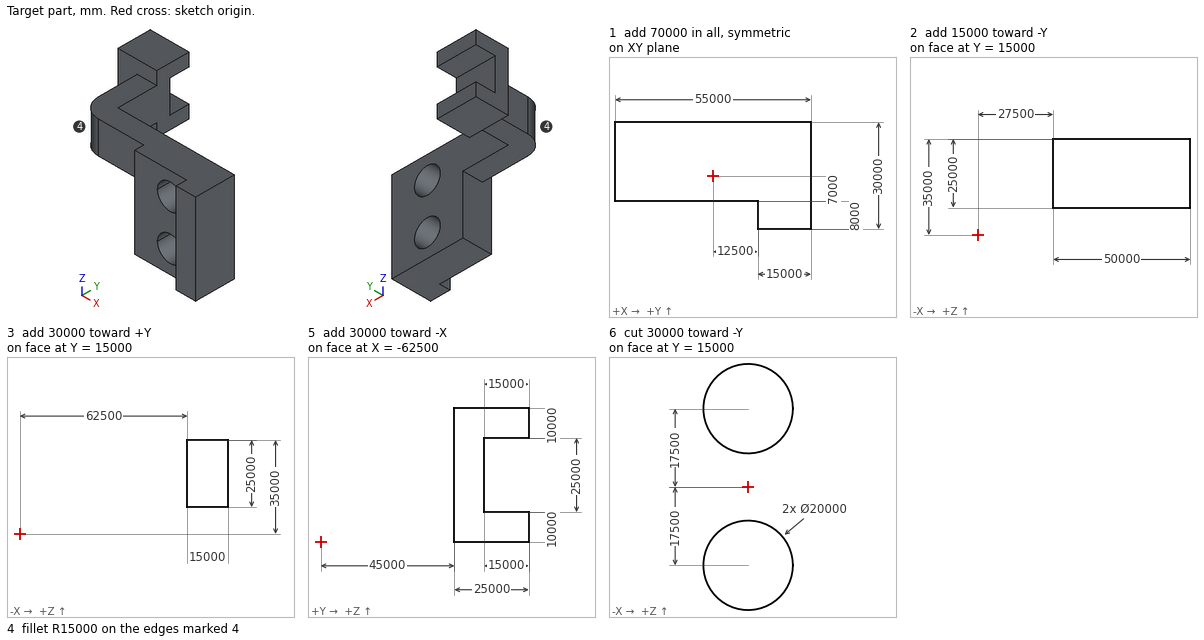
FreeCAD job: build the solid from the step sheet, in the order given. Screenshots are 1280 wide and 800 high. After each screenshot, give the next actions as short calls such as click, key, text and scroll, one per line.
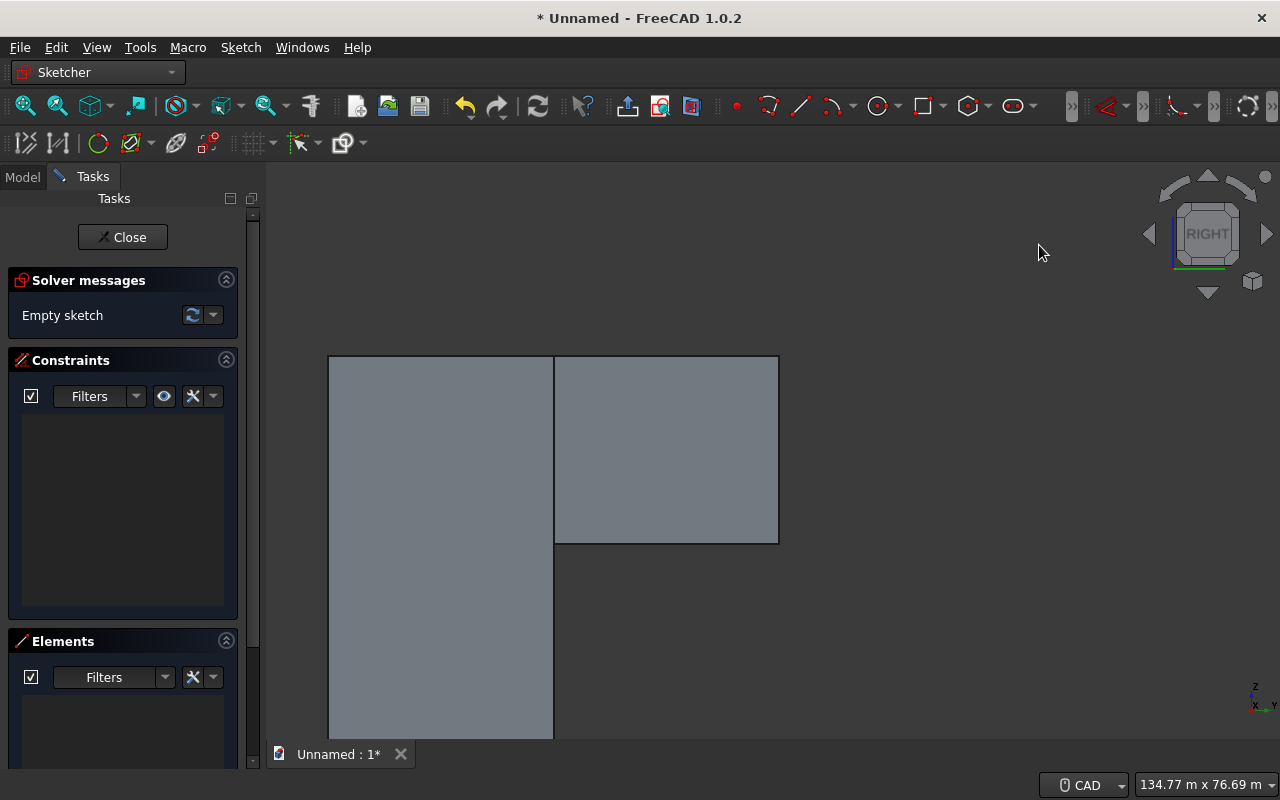
key(g)
key(m)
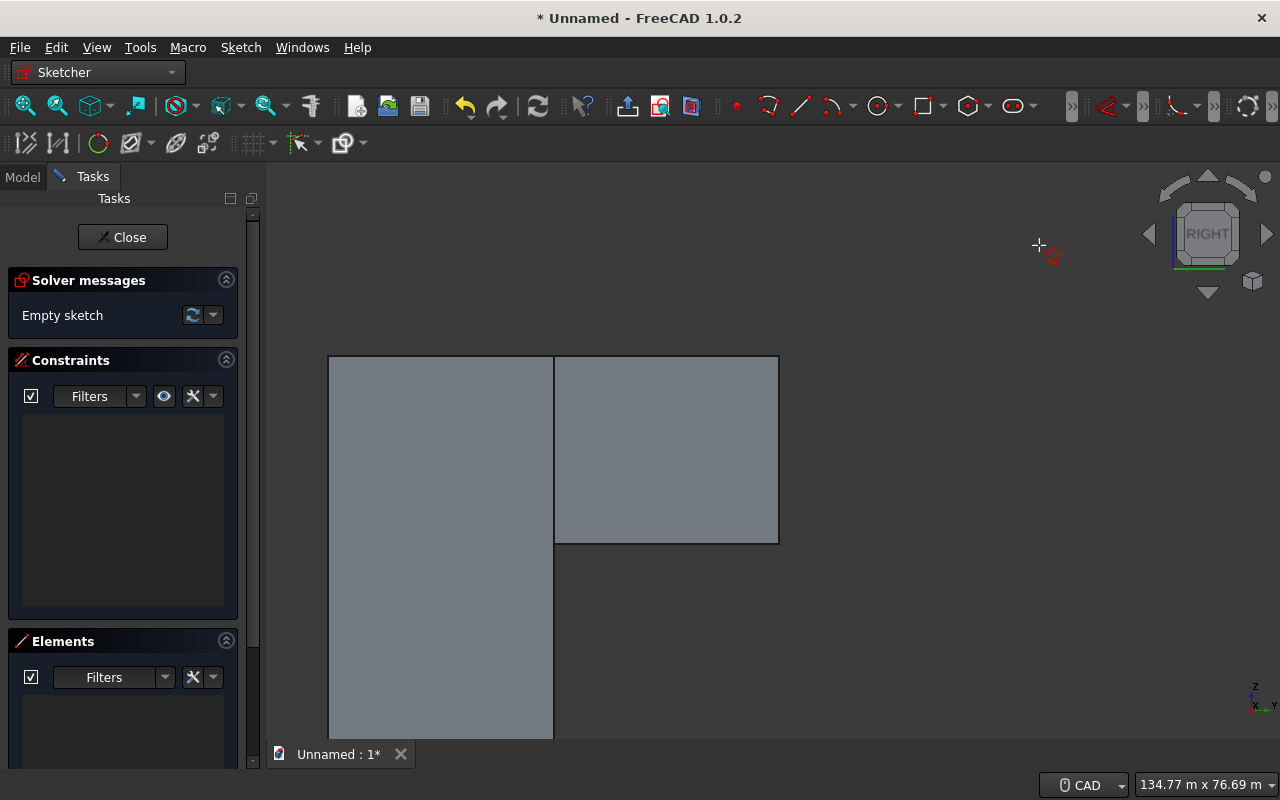
click(779, 619)
click(968, 610)
click(968, 544)
click(855, 544)
click(855, 356)
click(968, 356)
click(968, 281)
click(779, 281)
click(779, 620)
key(Escape)
key(Escape)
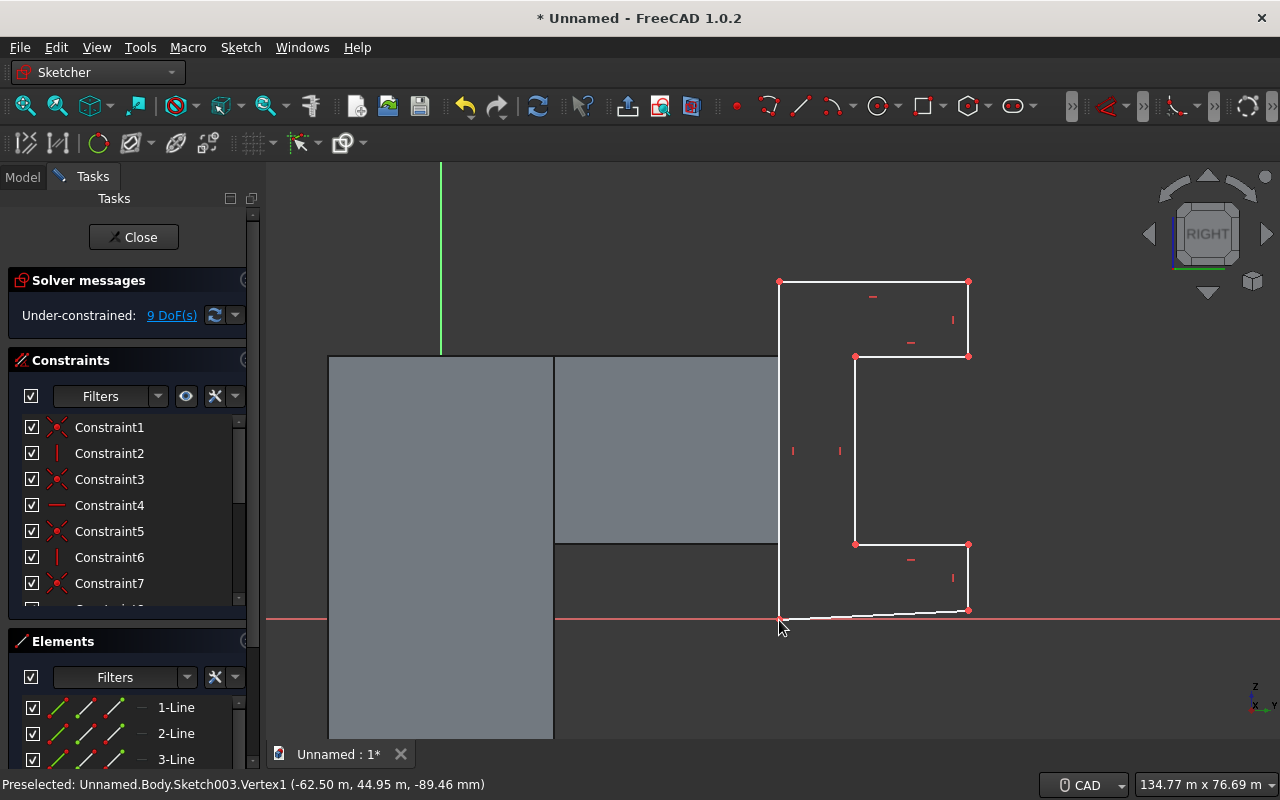
click(836, 617)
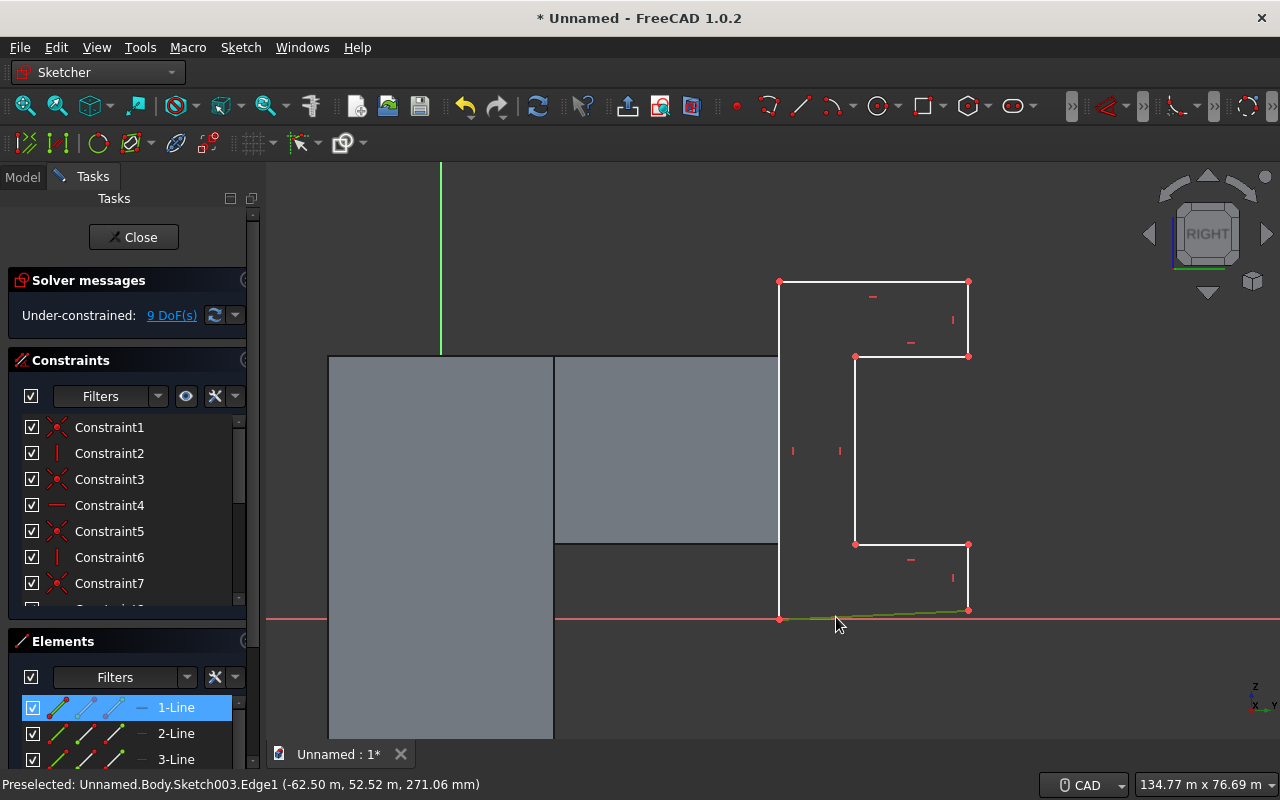
key(h)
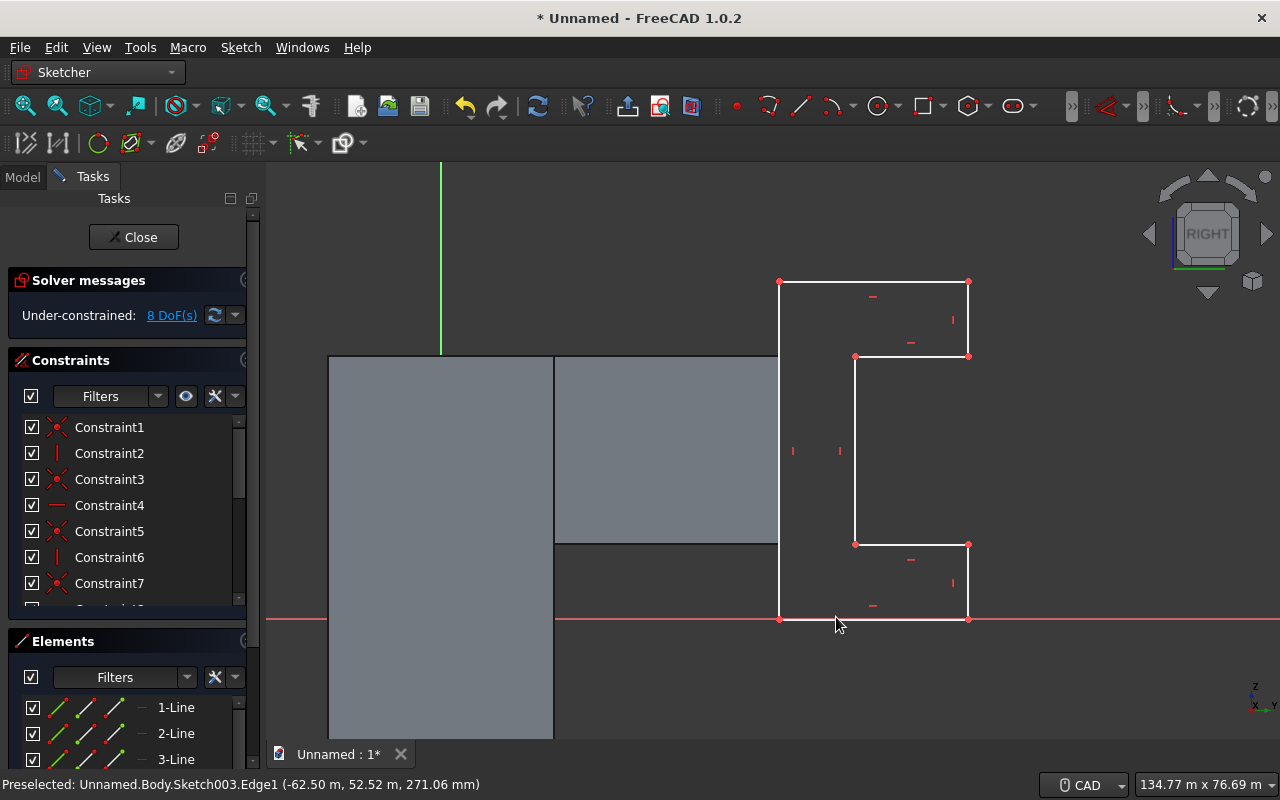
click(779, 620)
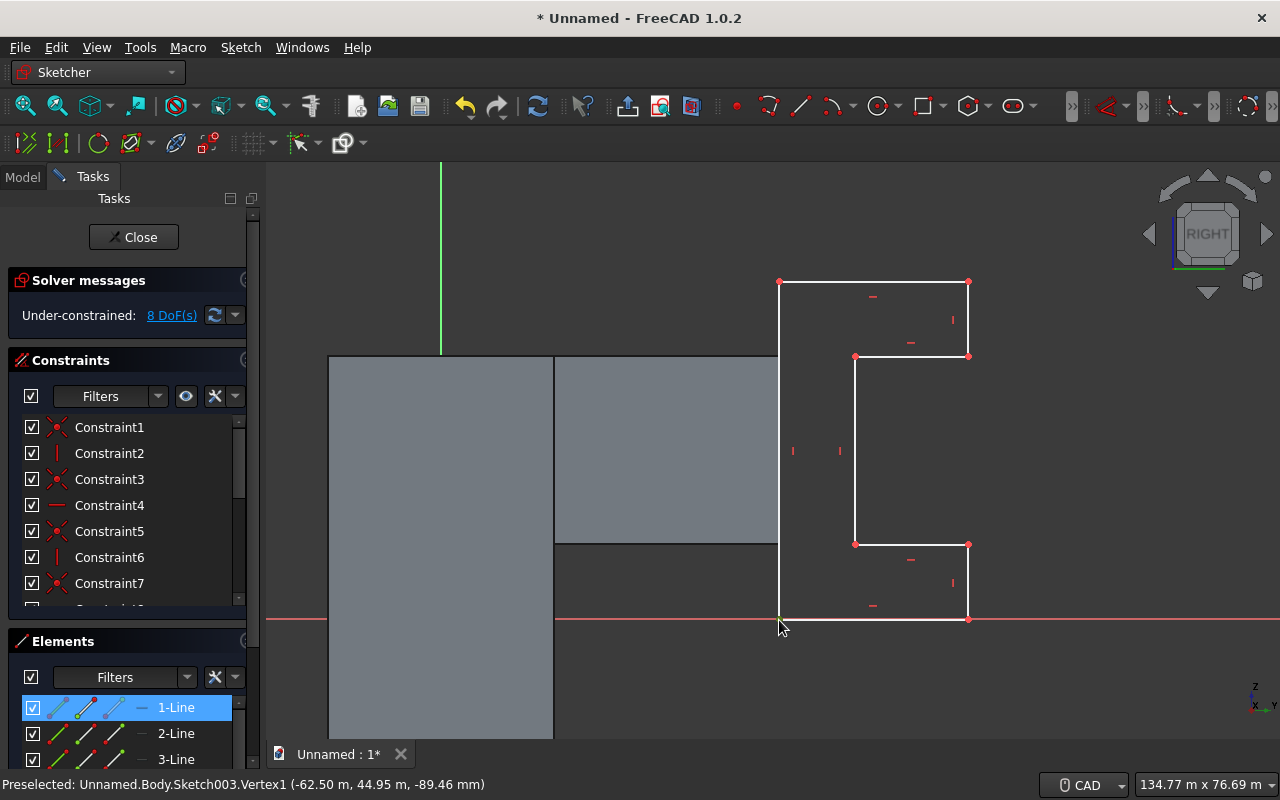
click(353, 619)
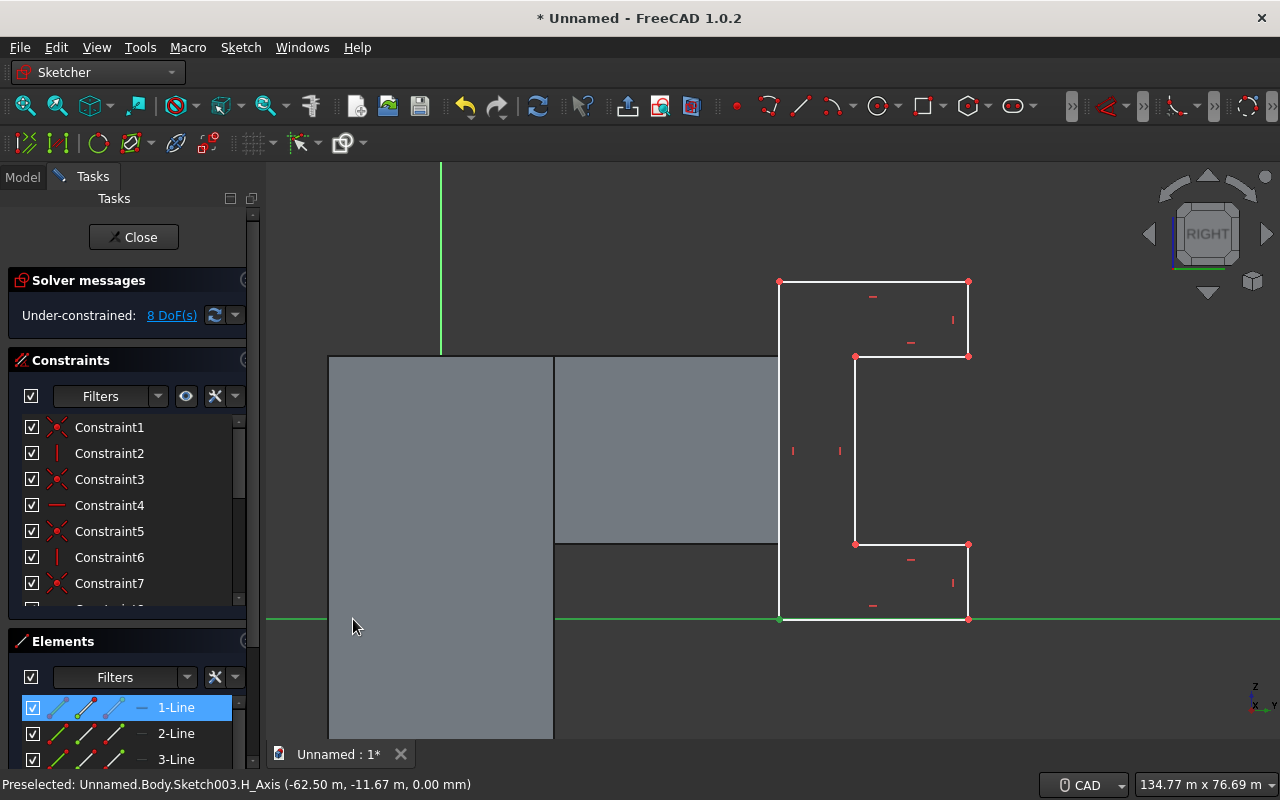
key(c)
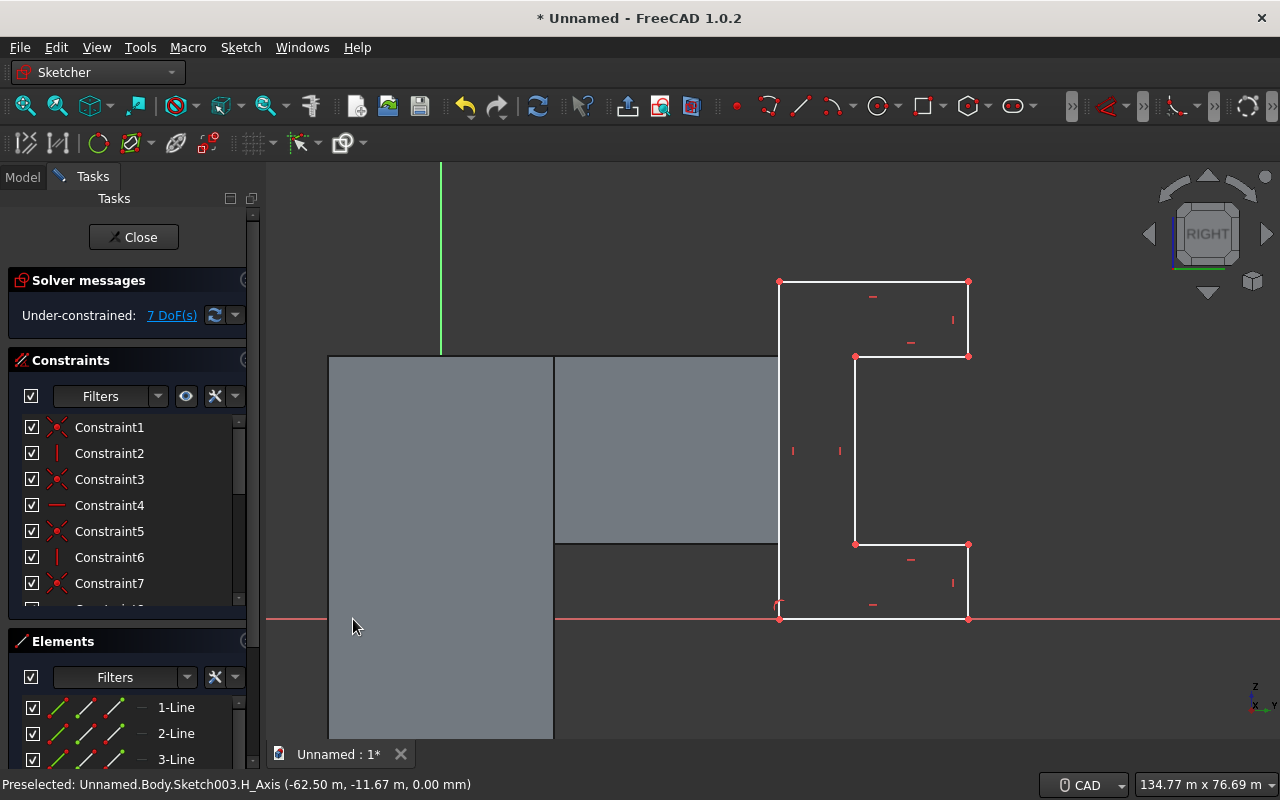
key(d)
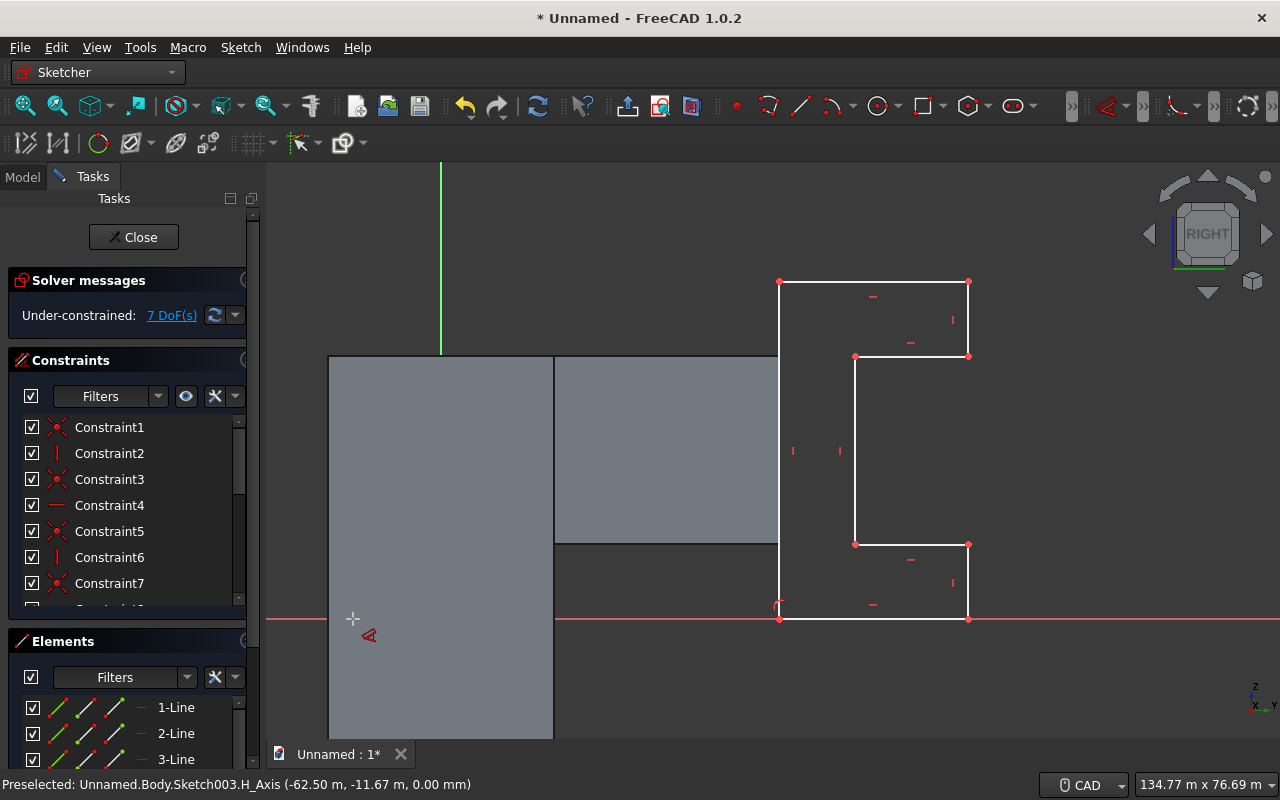
click(836, 619)
click(874, 653)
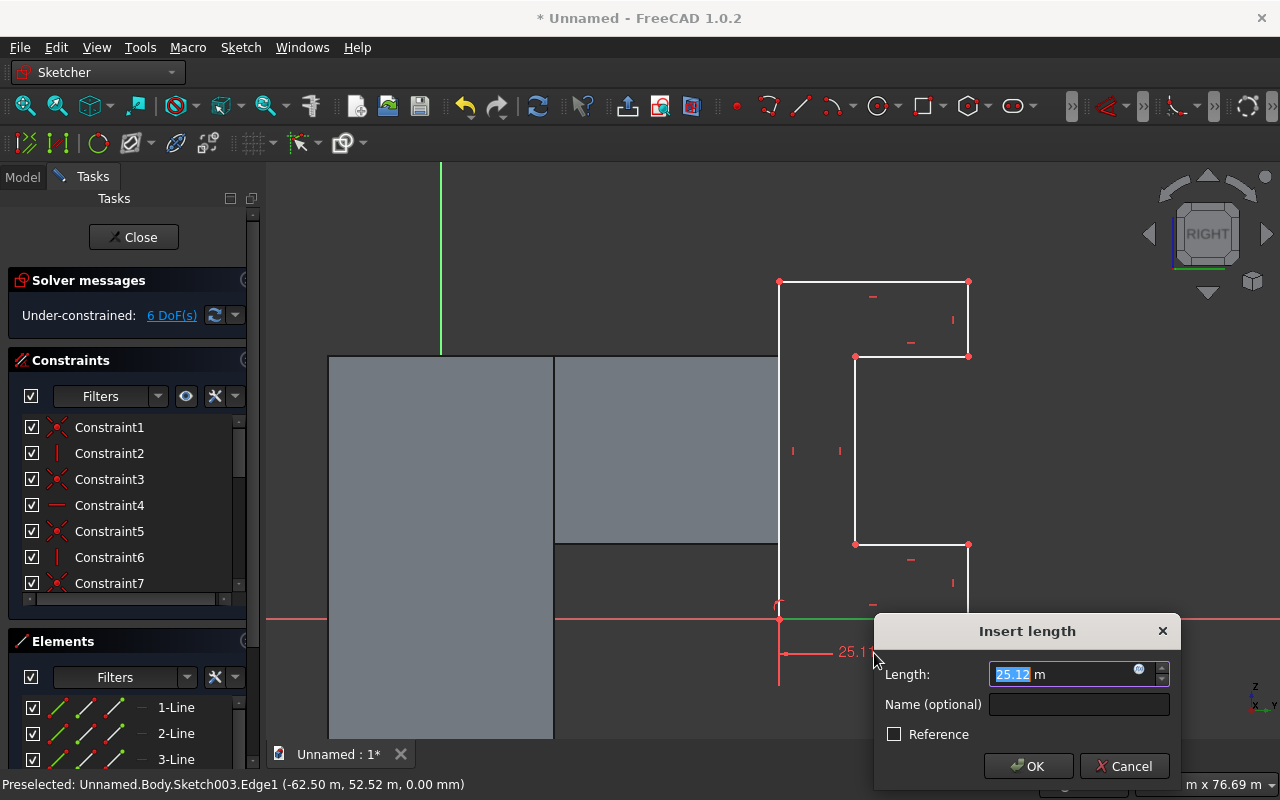
key(ctrl+a)
text(25000 mm)
key(Return)